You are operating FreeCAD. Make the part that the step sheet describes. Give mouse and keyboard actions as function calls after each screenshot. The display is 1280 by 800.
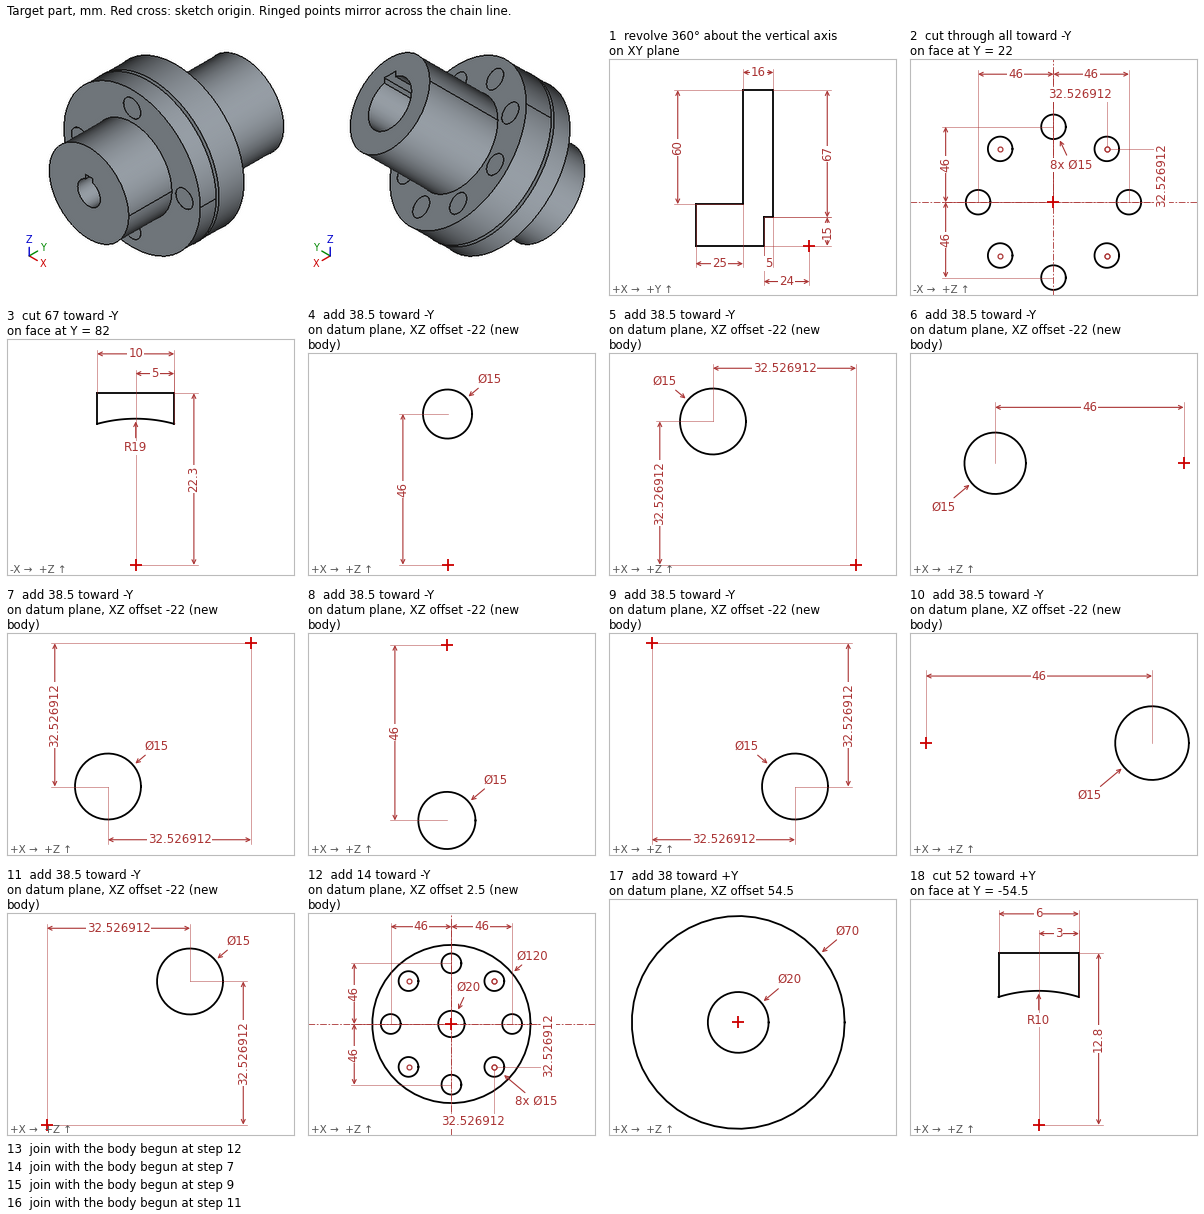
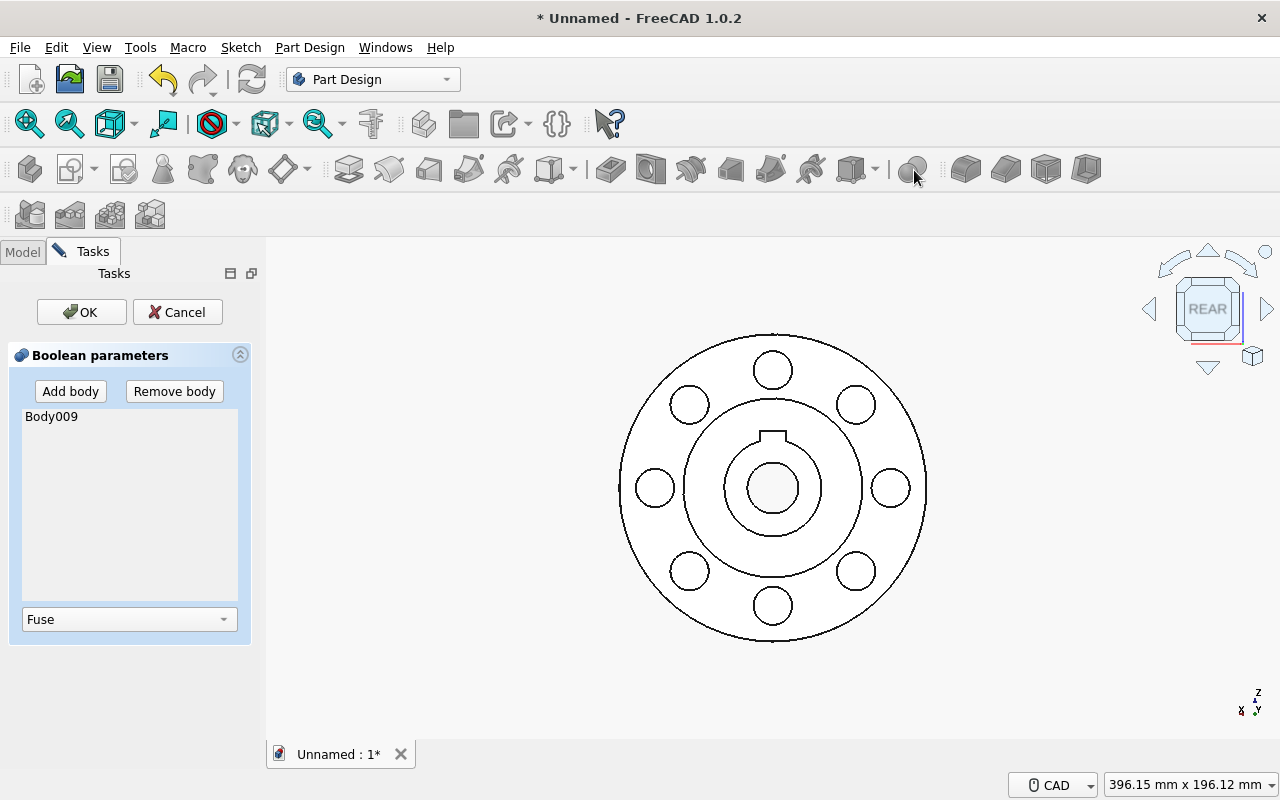
click(82, 312)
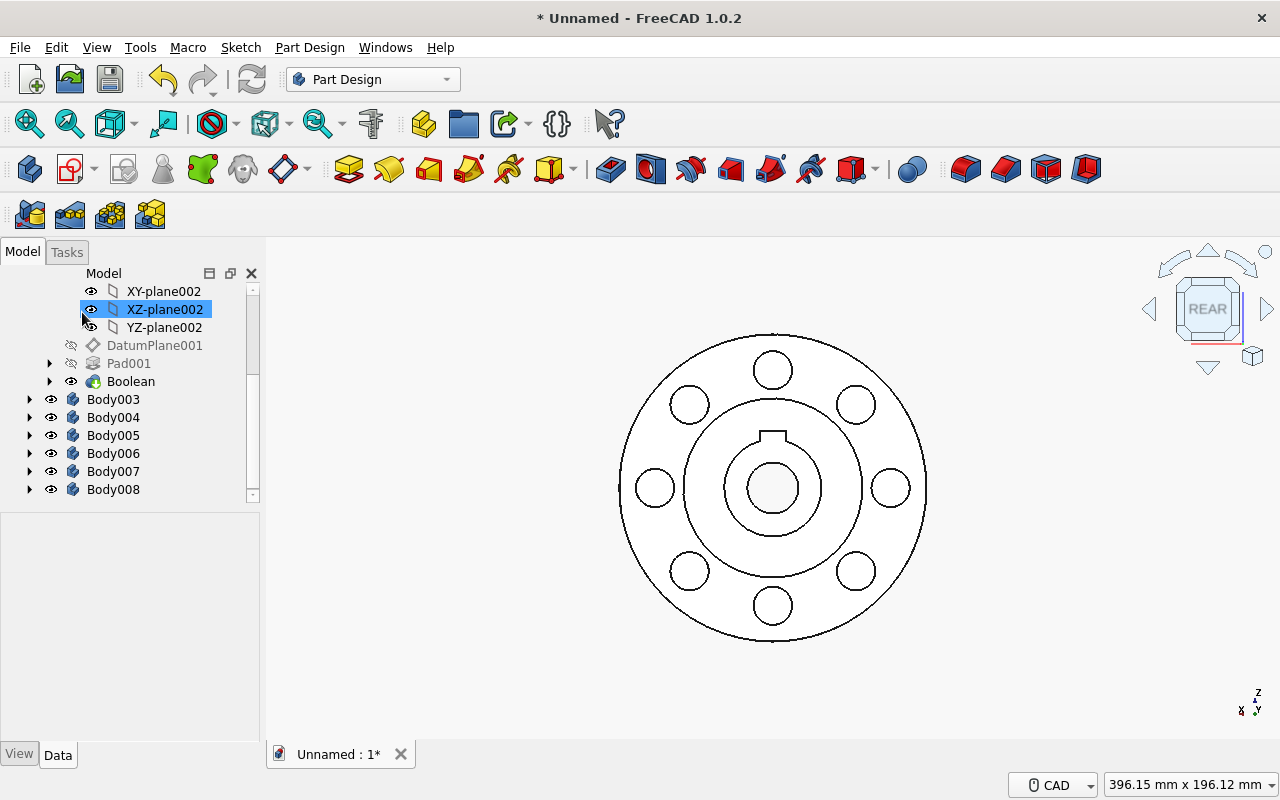
click(96, 417)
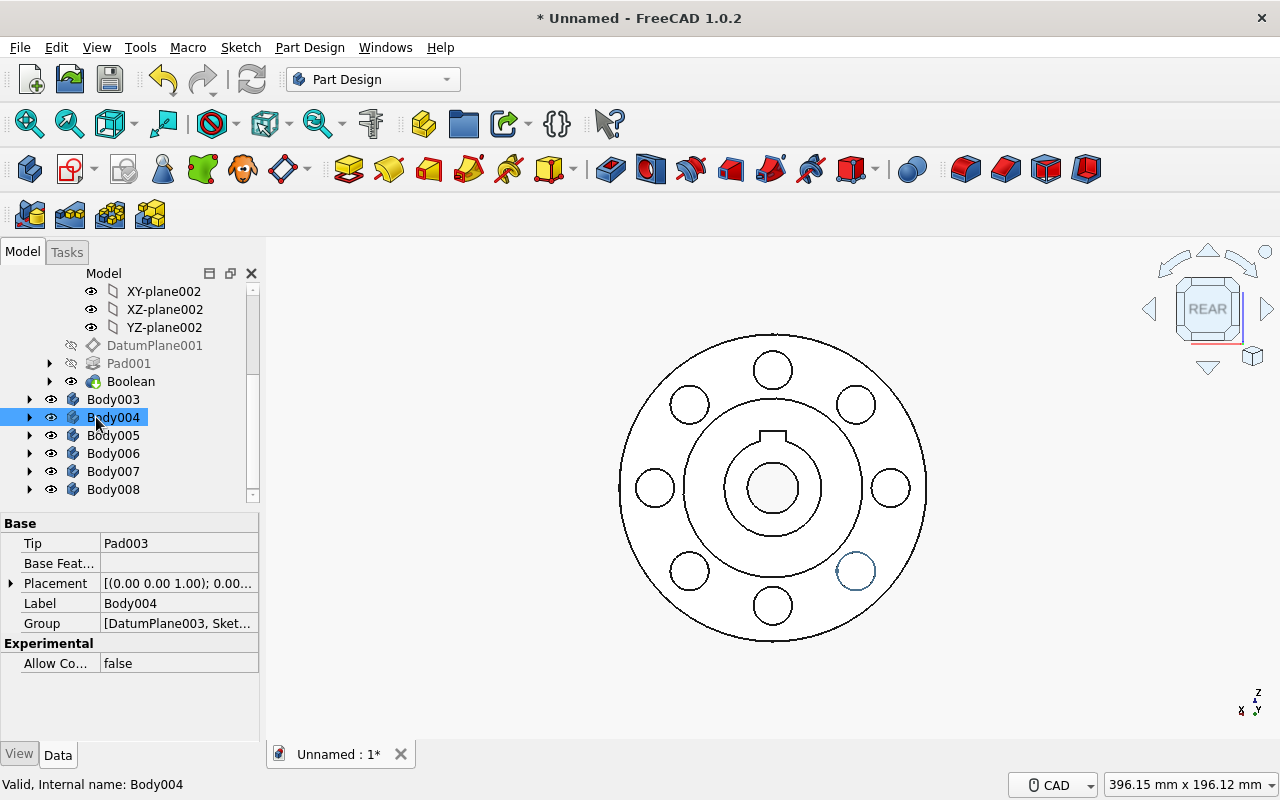
click(914, 170)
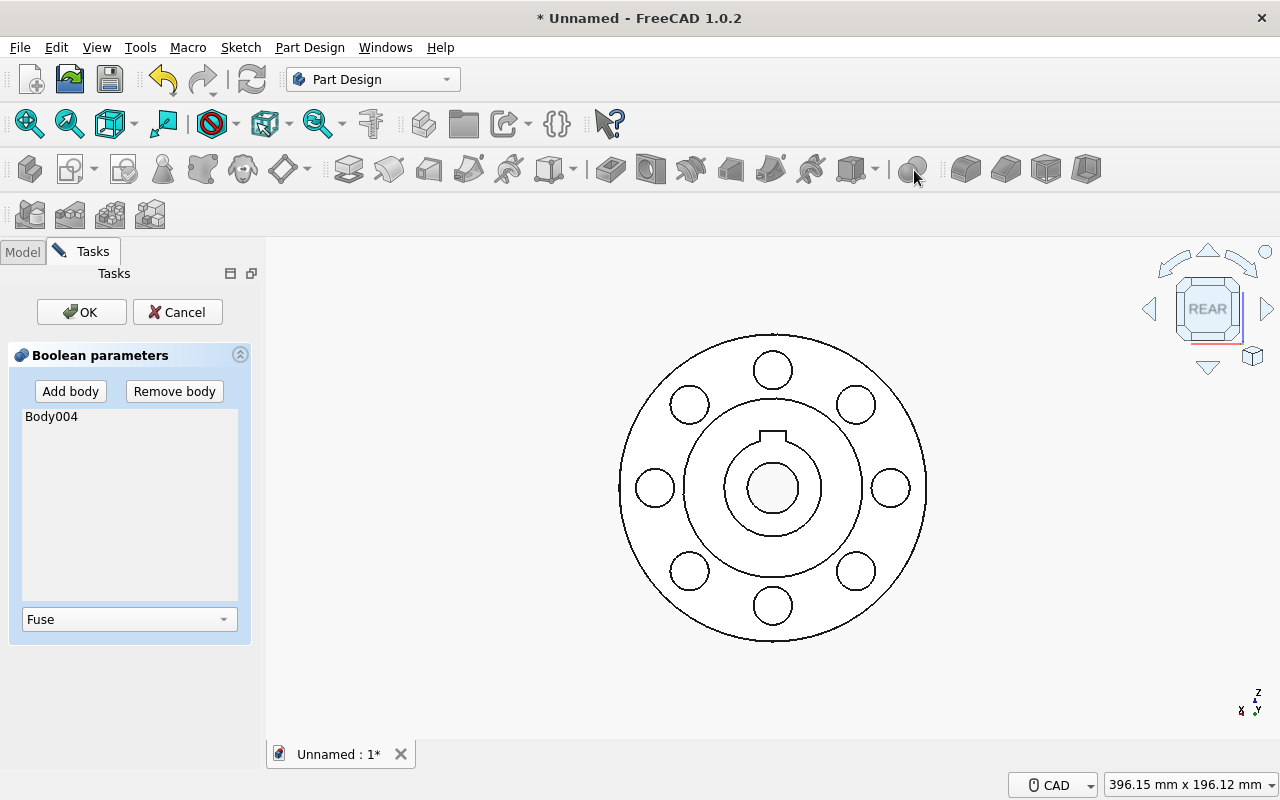
click(82, 312)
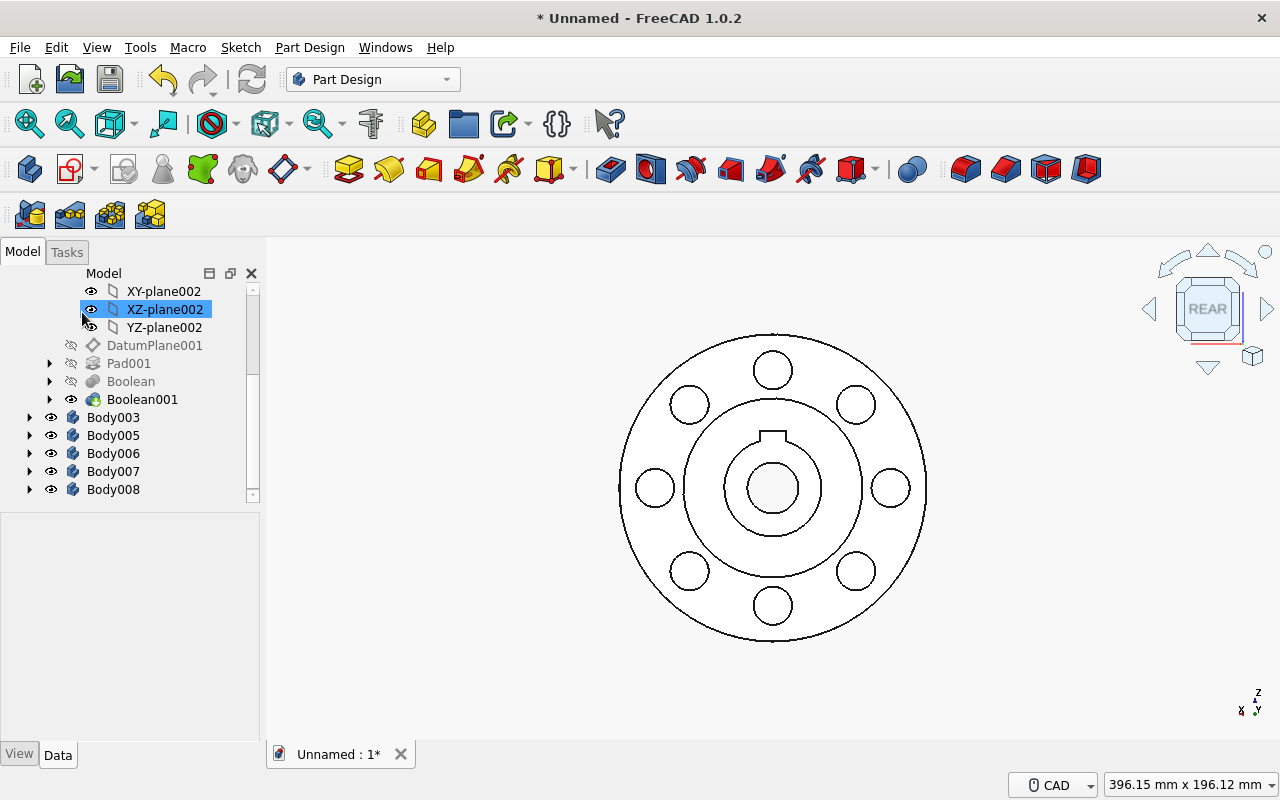
click(96, 453)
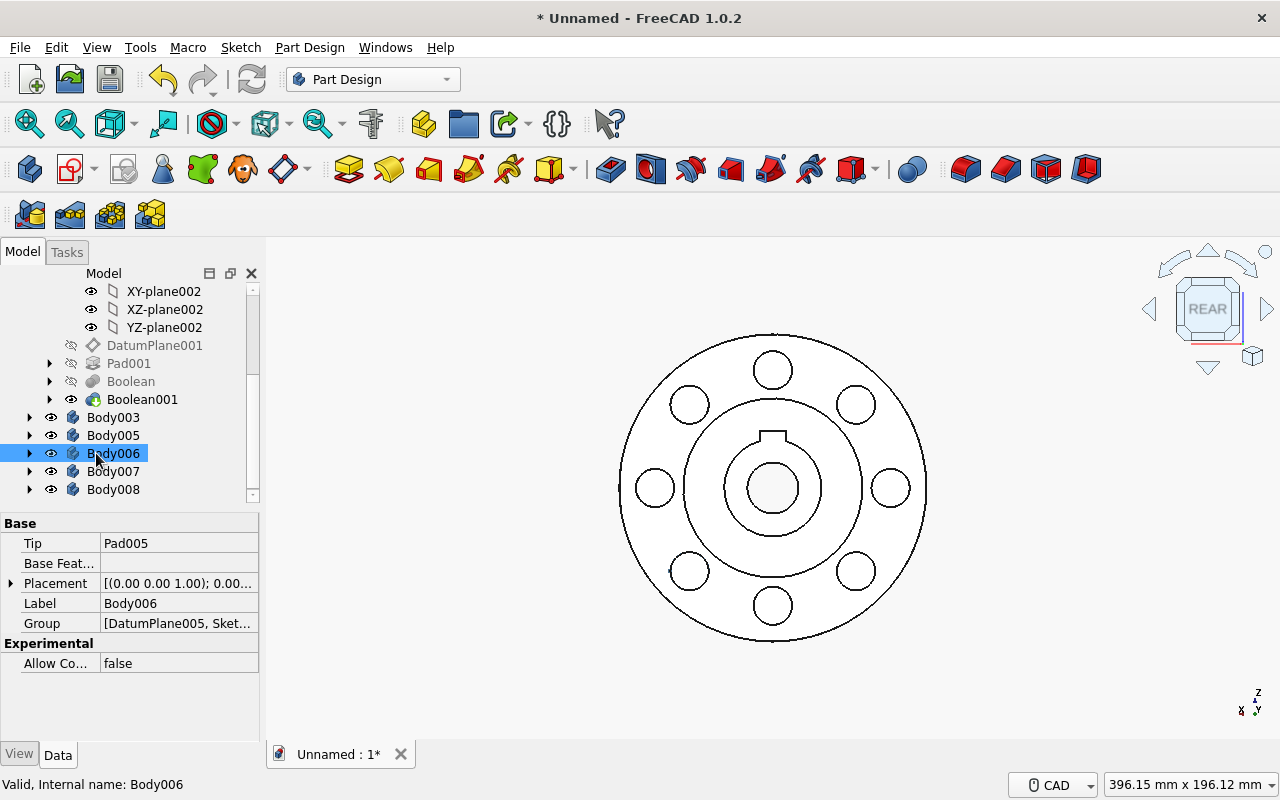
click(914, 170)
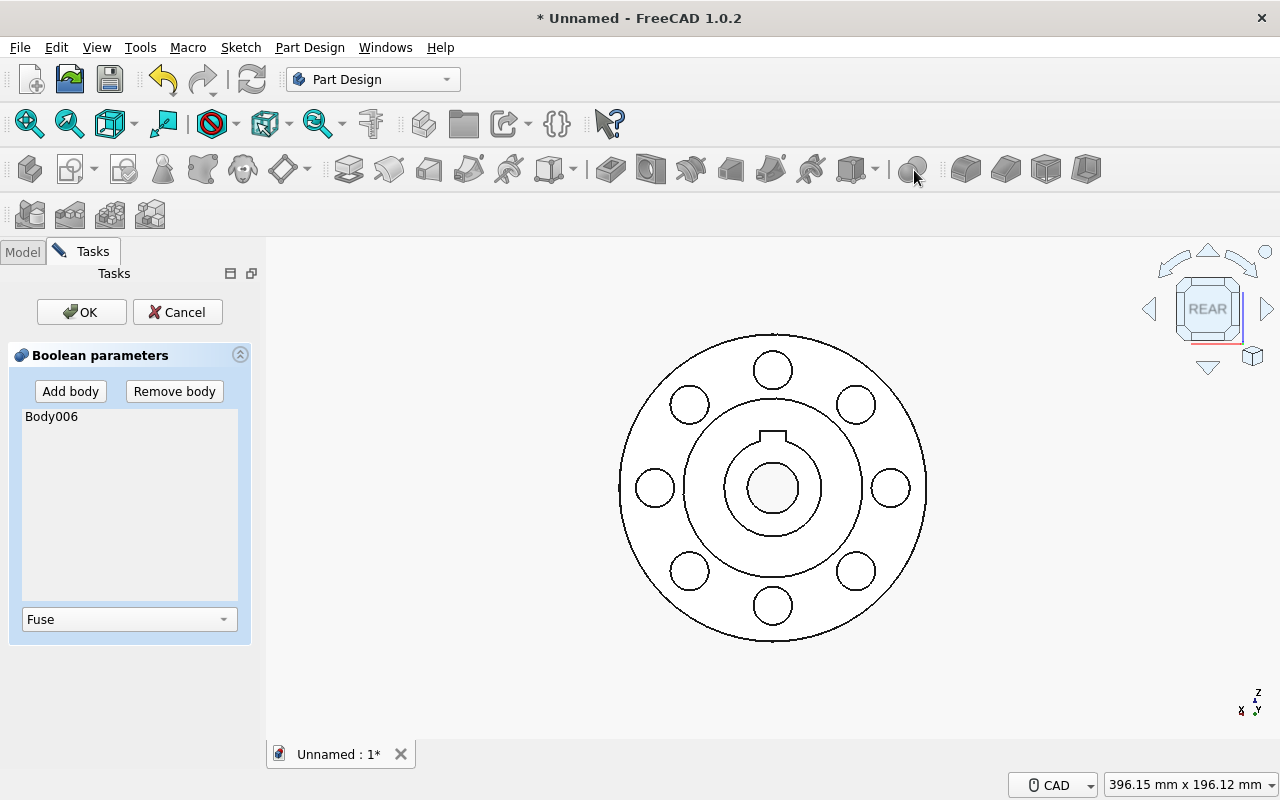
click(82, 312)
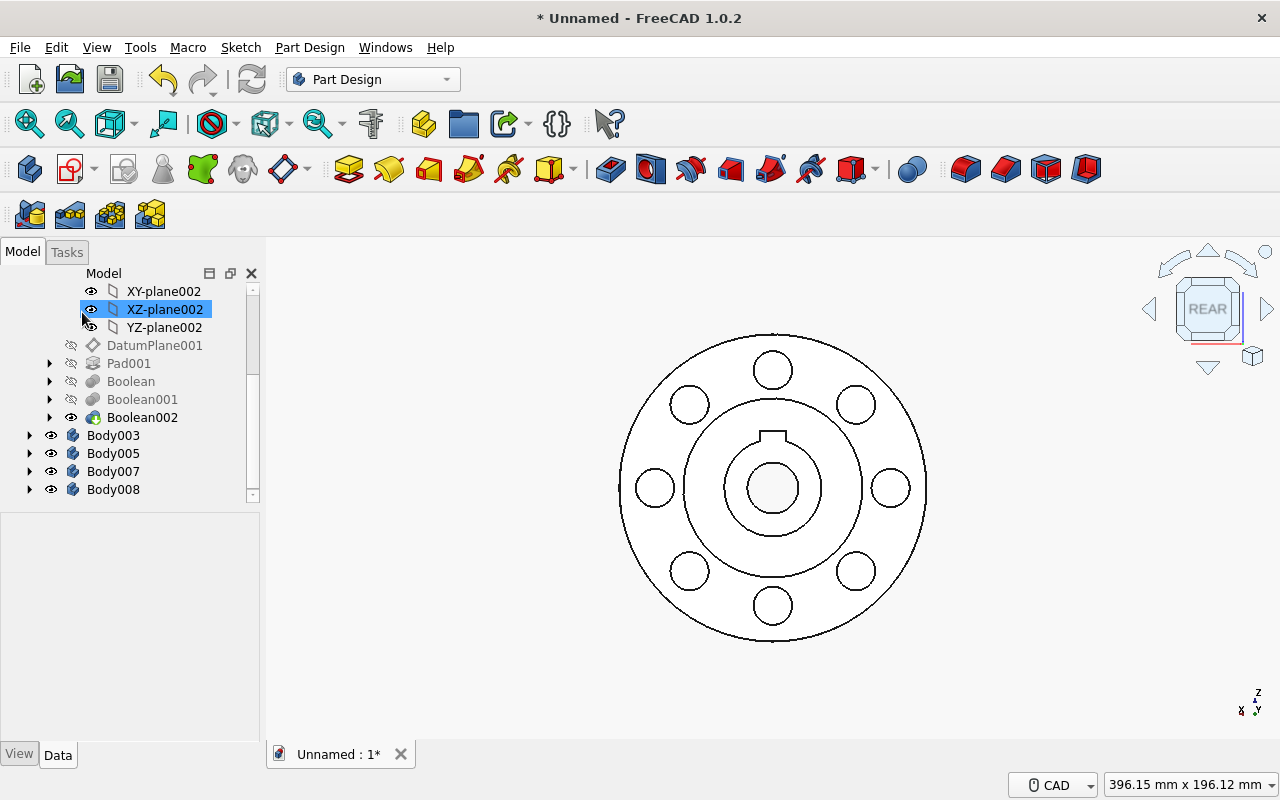
click(96, 489)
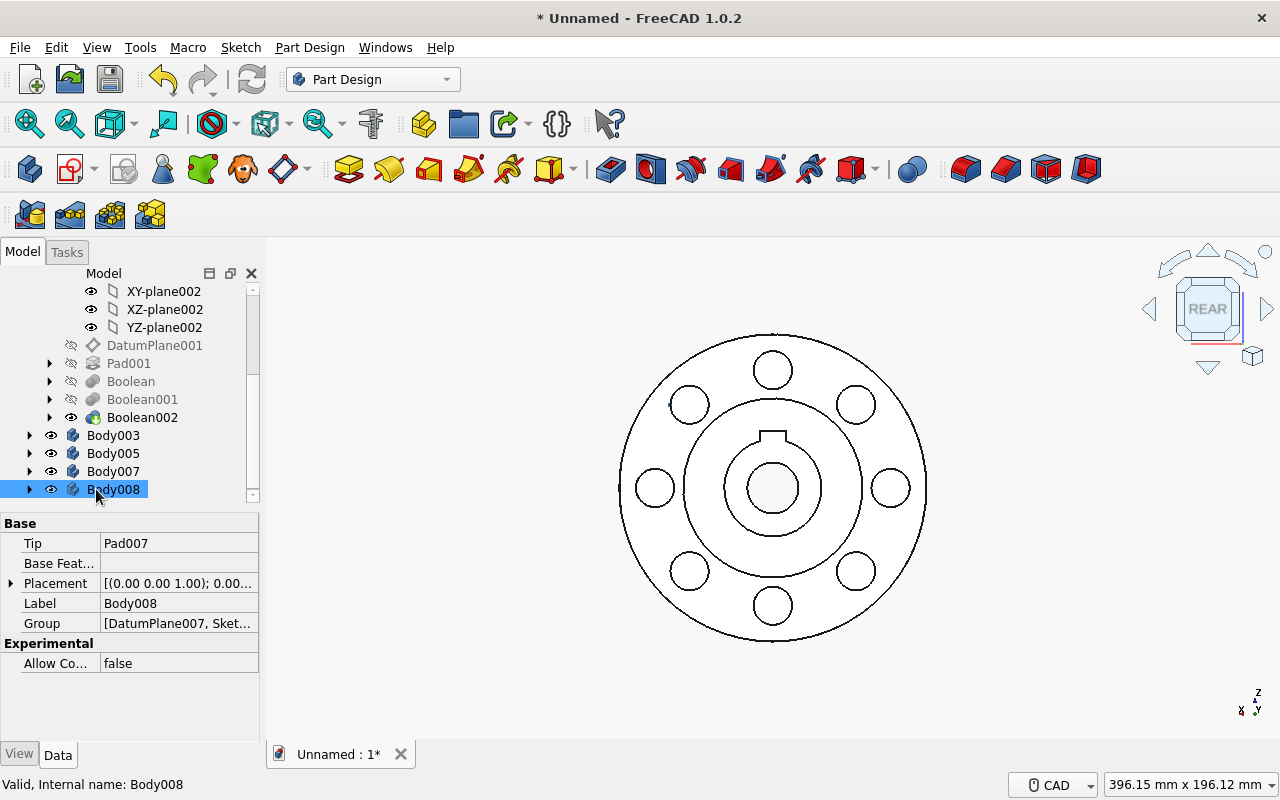
click(914, 170)